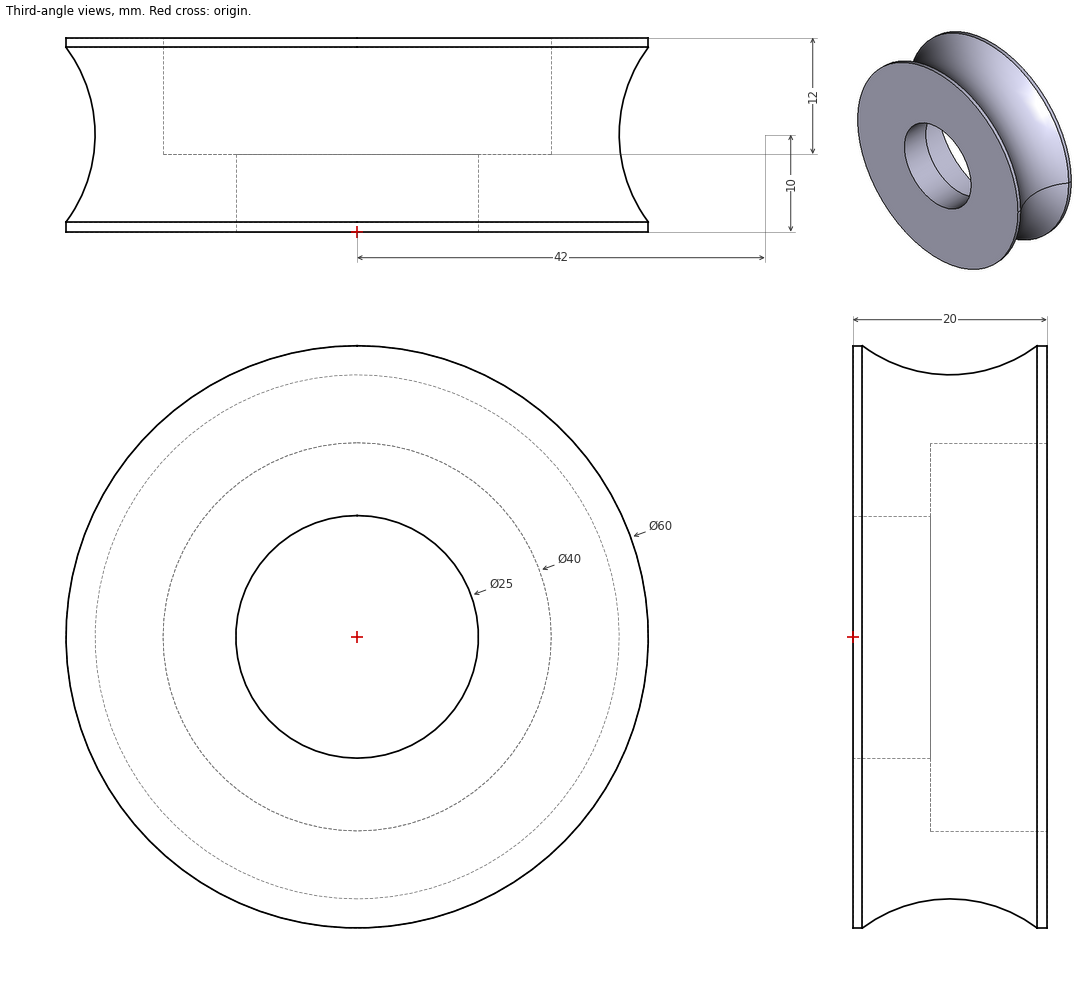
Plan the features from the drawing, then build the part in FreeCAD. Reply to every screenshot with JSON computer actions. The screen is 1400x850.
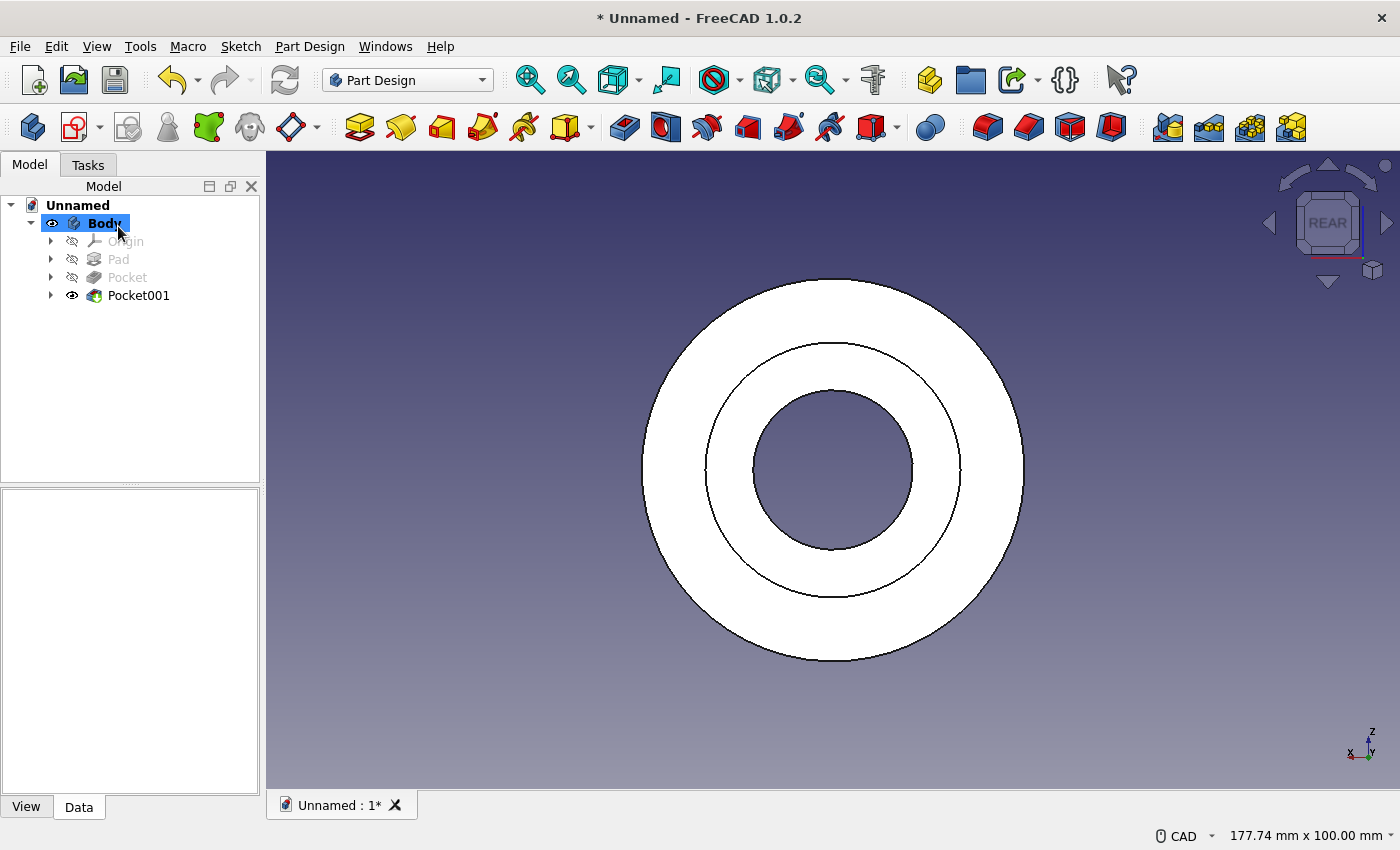
{"action": "left_click", "coordinate": [74, 128]}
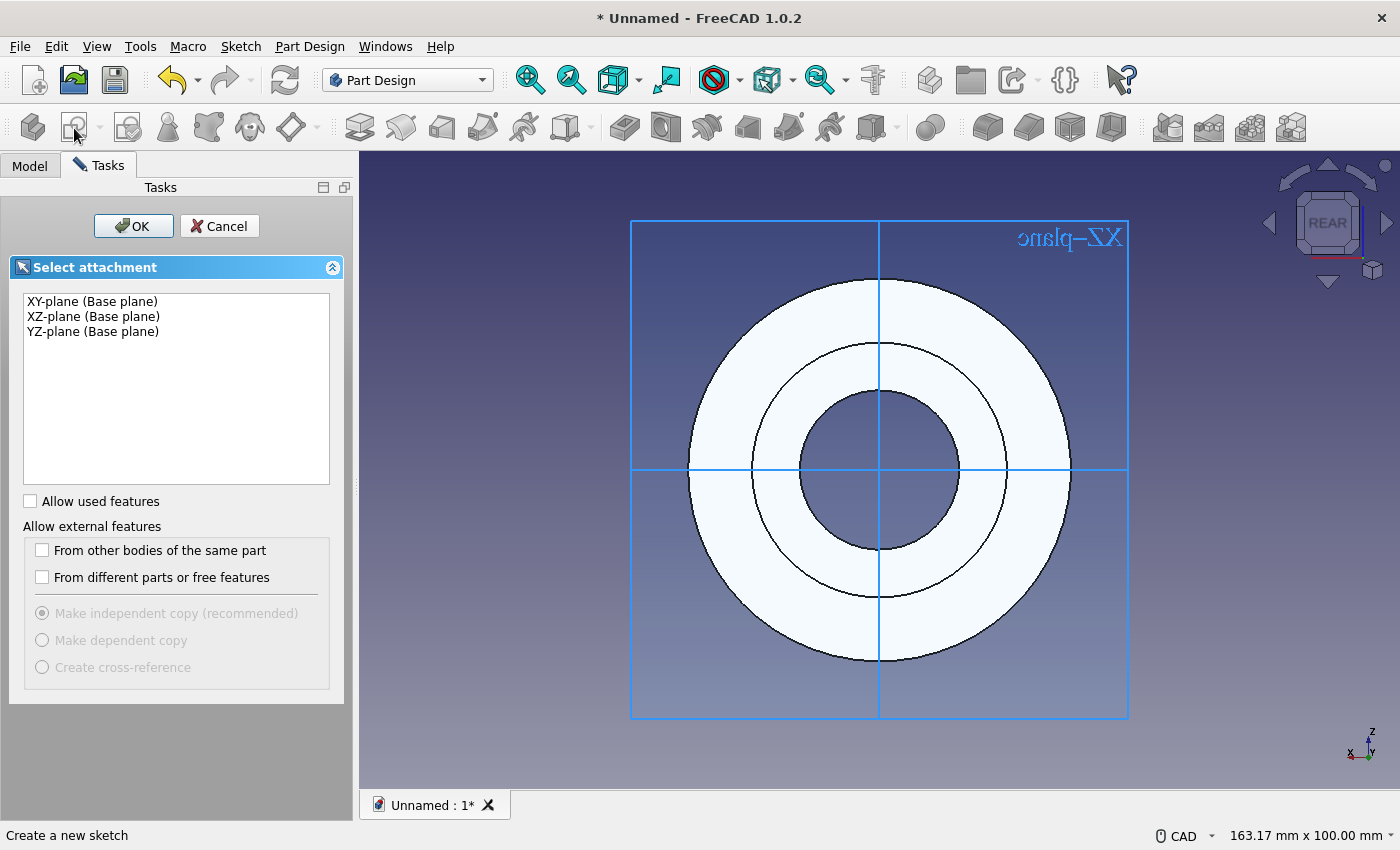
{"action": "left_click", "coordinate": [84, 302]}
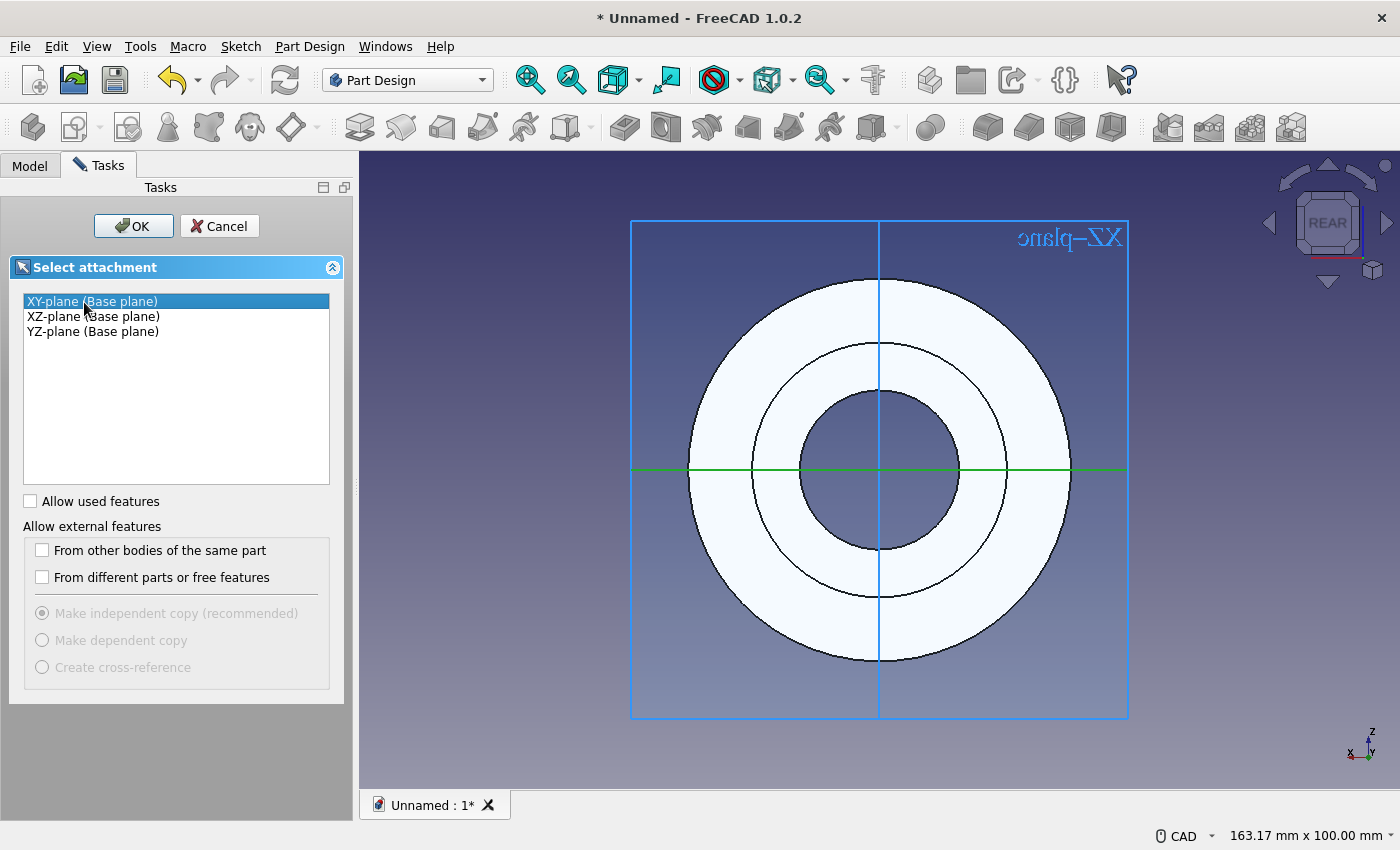
{"action": "left_click", "coordinate": [134, 226]}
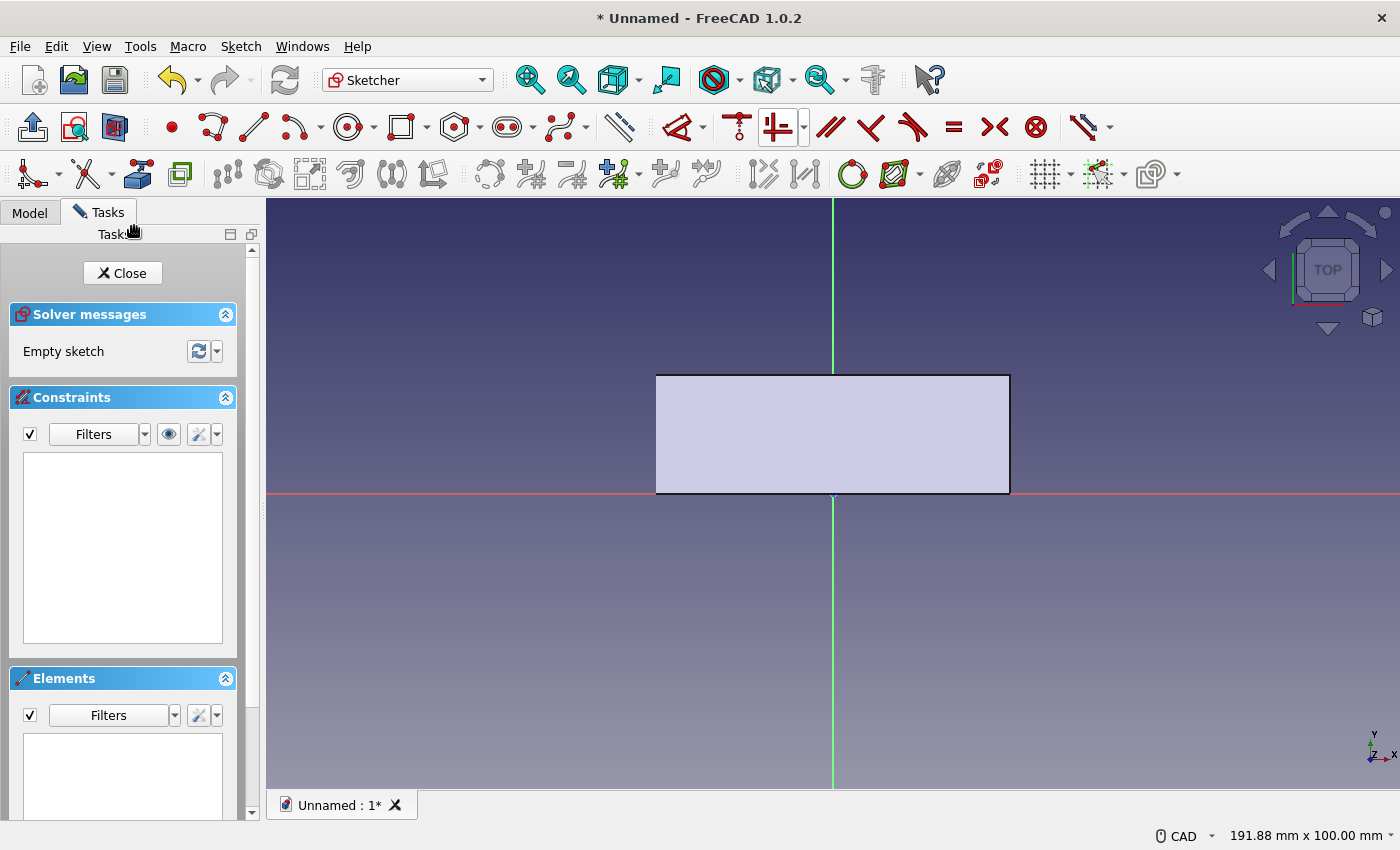
{"action": "left_click", "coordinate": [115, 128]}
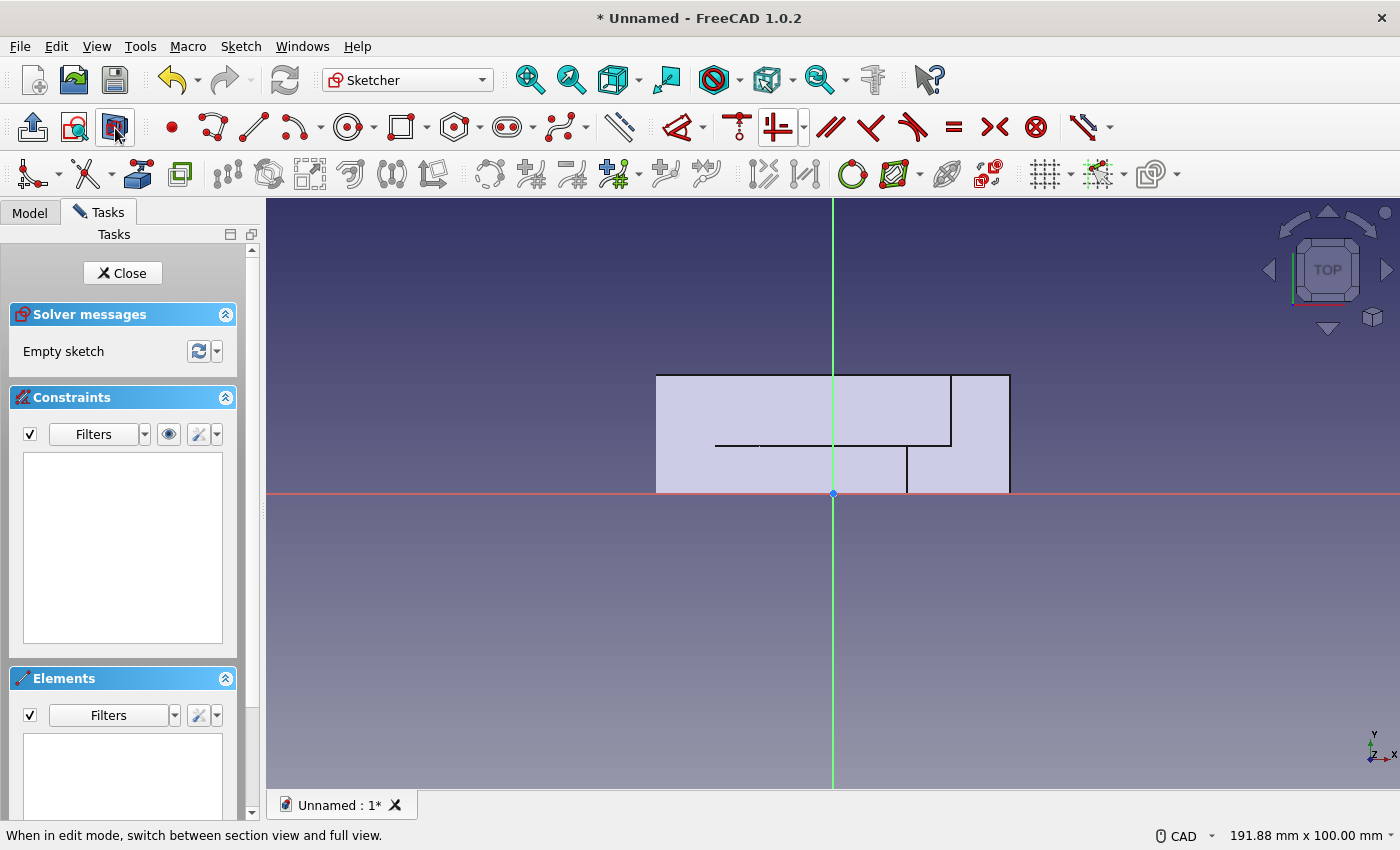
{"action": "scroll", "coordinate": [1235, 363], "scroll_direction": "up", "scroll_amount": 3}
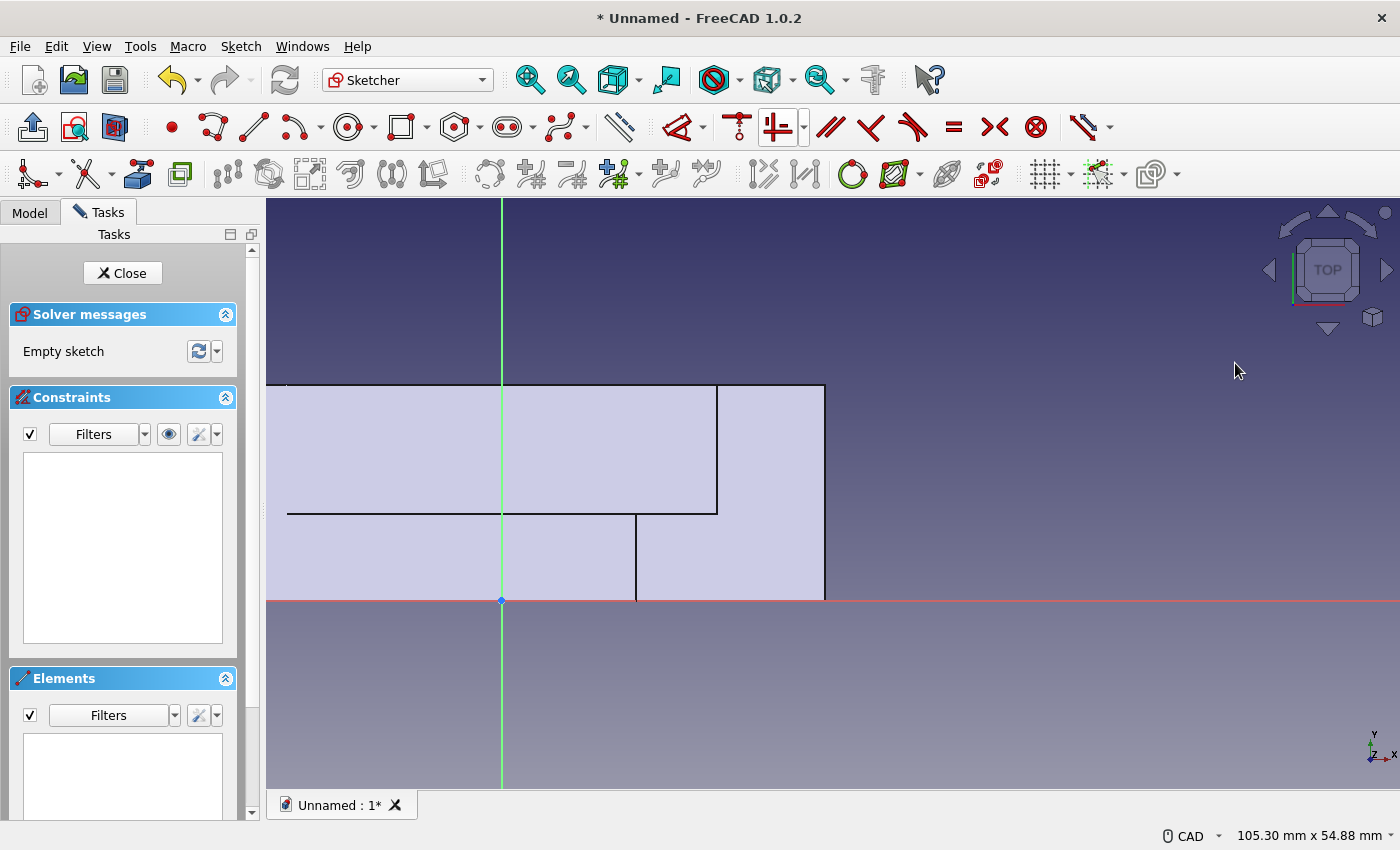
{"action": "left_click", "coordinate": [348, 128]}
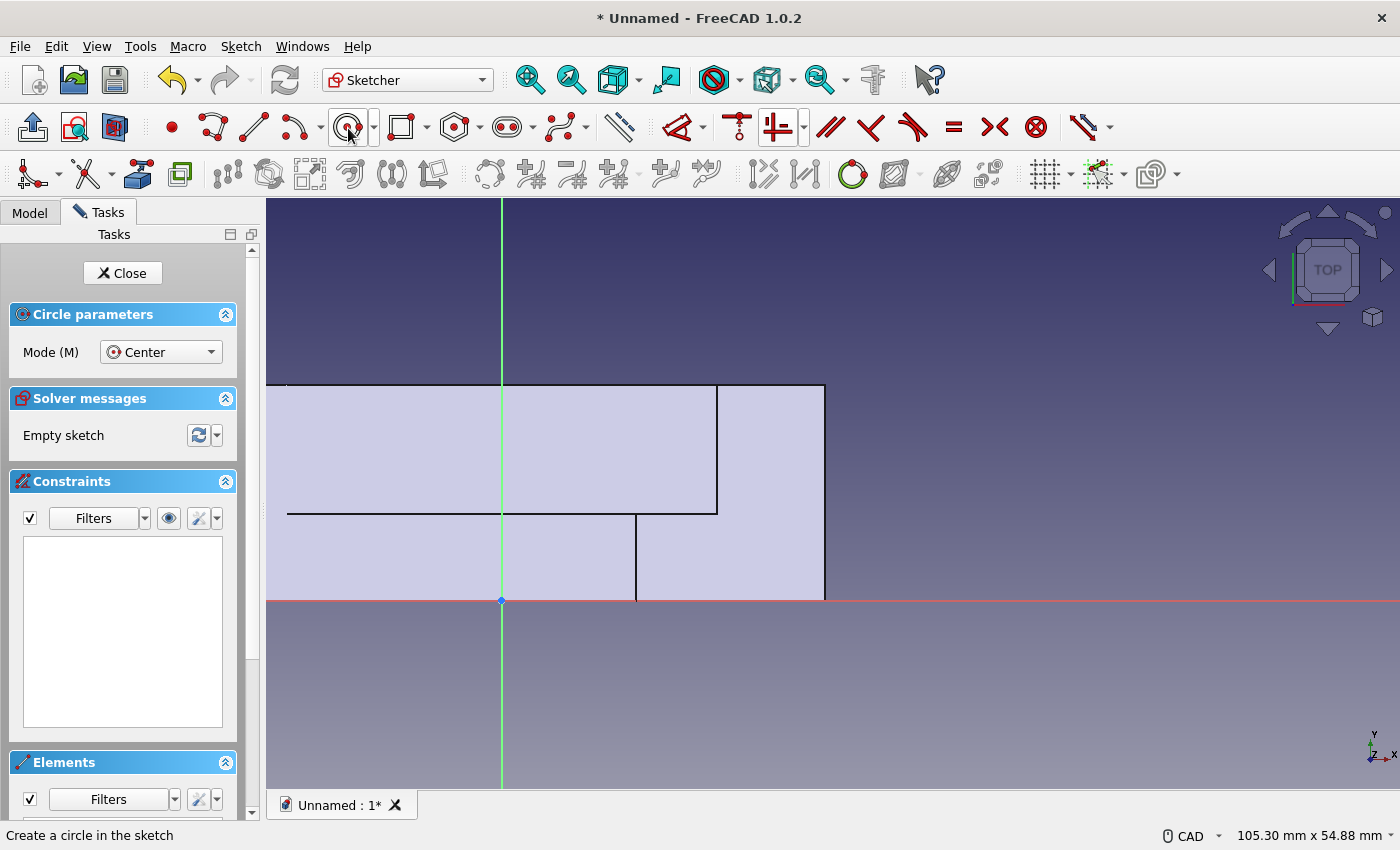
{"action": "left_click", "coordinate": [954, 493]}
{"action": "left_click", "coordinate": [1068, 379]}
{"action": "key", "text": "Escape"}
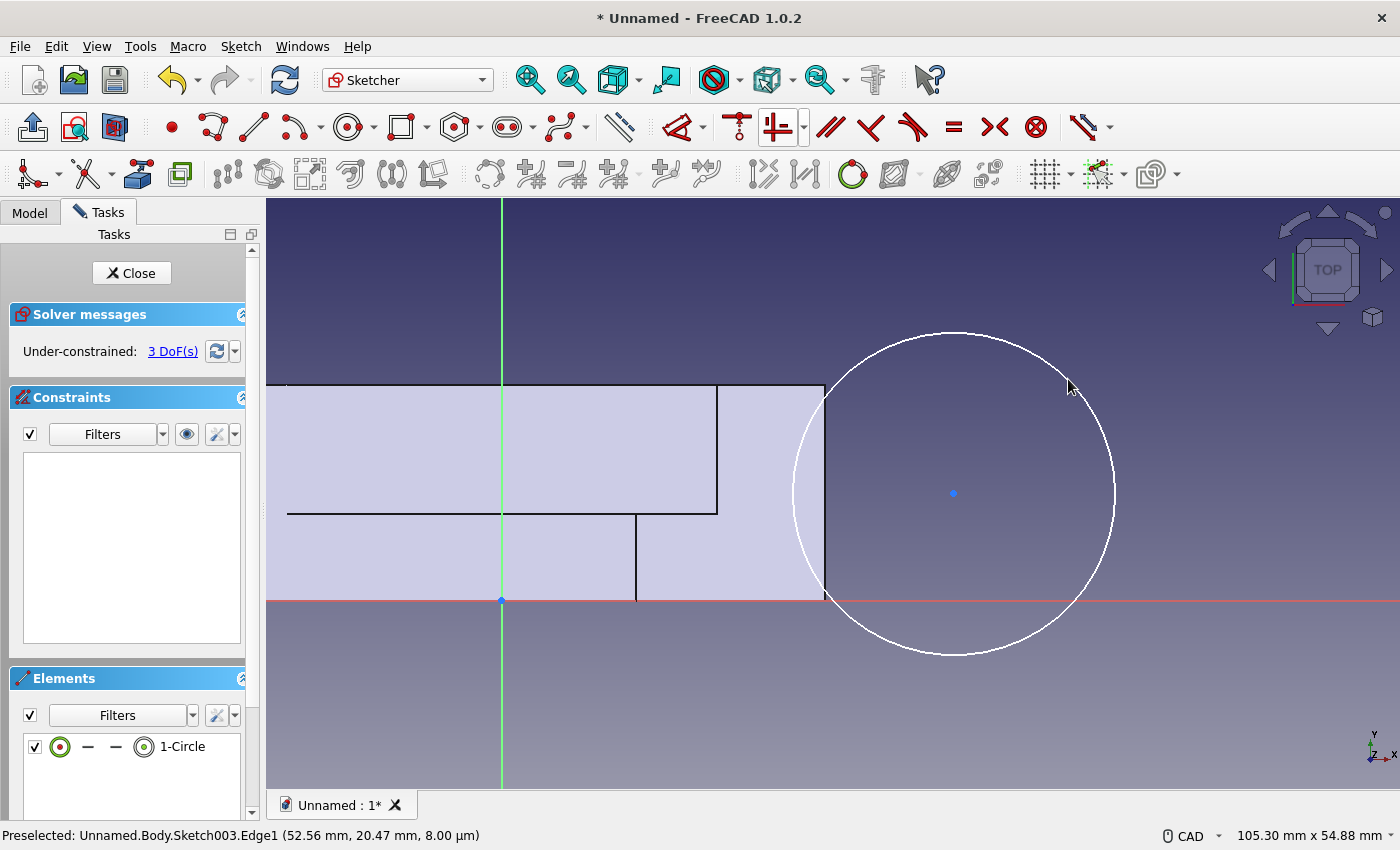
{"action": "left_click", "coordinate": [676, 128]}